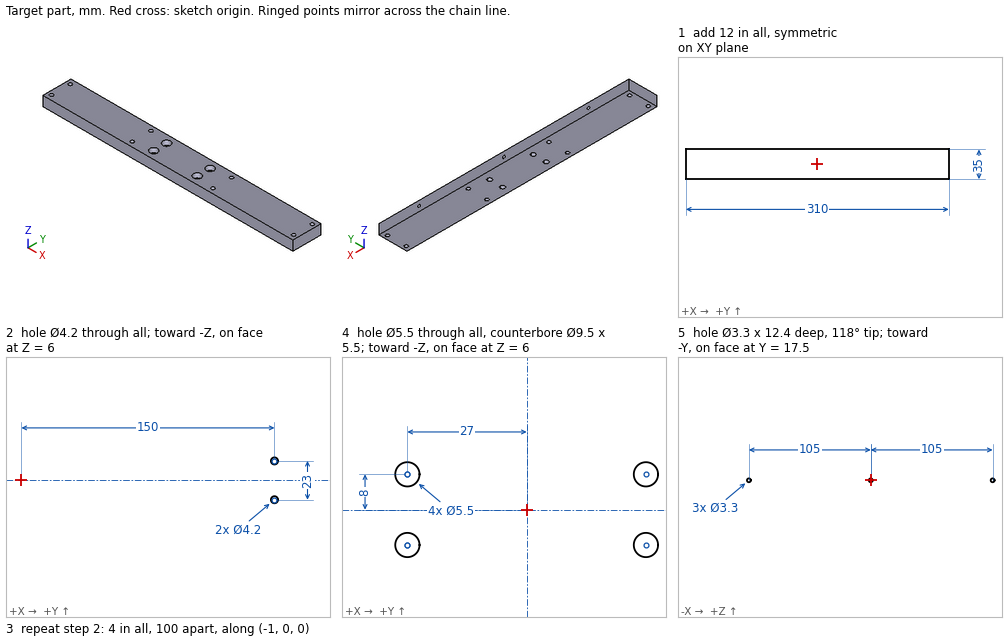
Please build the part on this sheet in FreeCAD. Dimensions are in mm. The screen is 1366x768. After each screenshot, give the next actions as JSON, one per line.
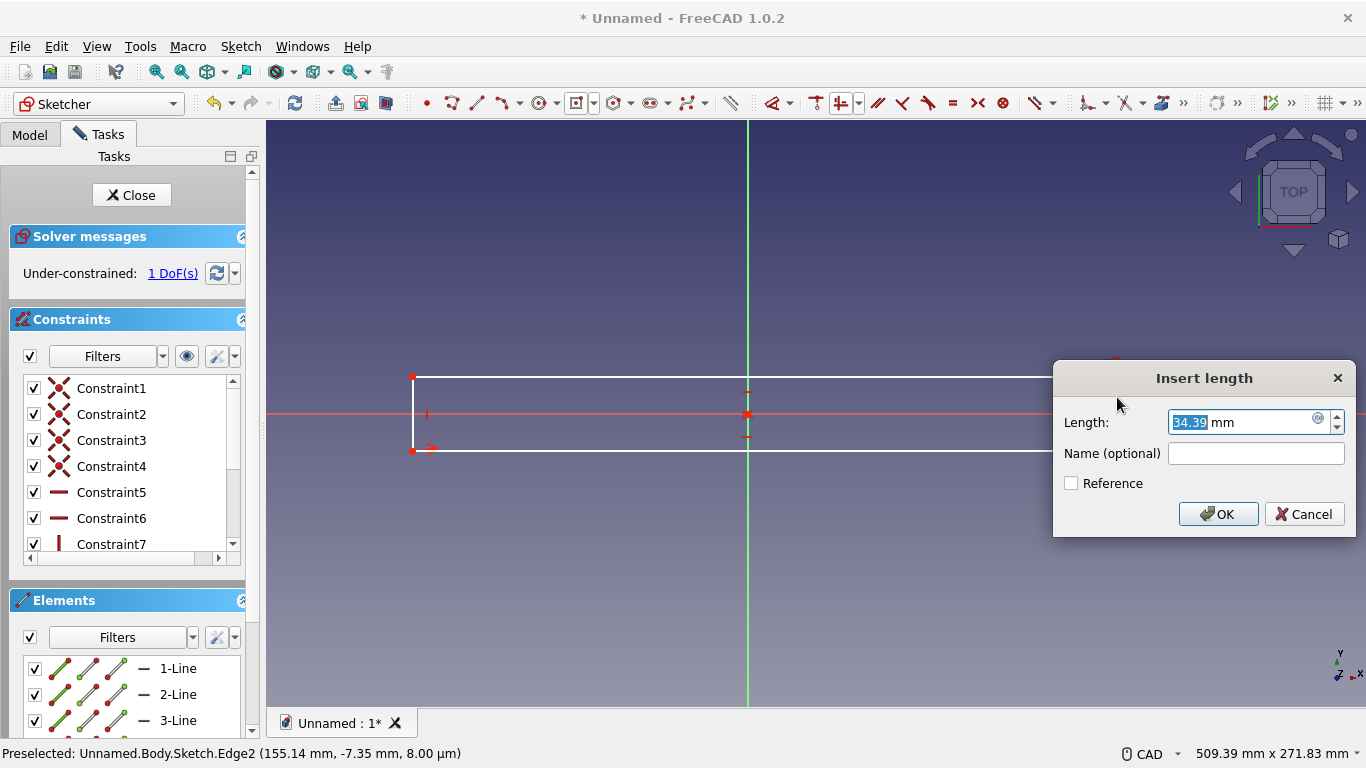
{"action": "type", "text": "35"}
{"action": "key", "text": "Return"}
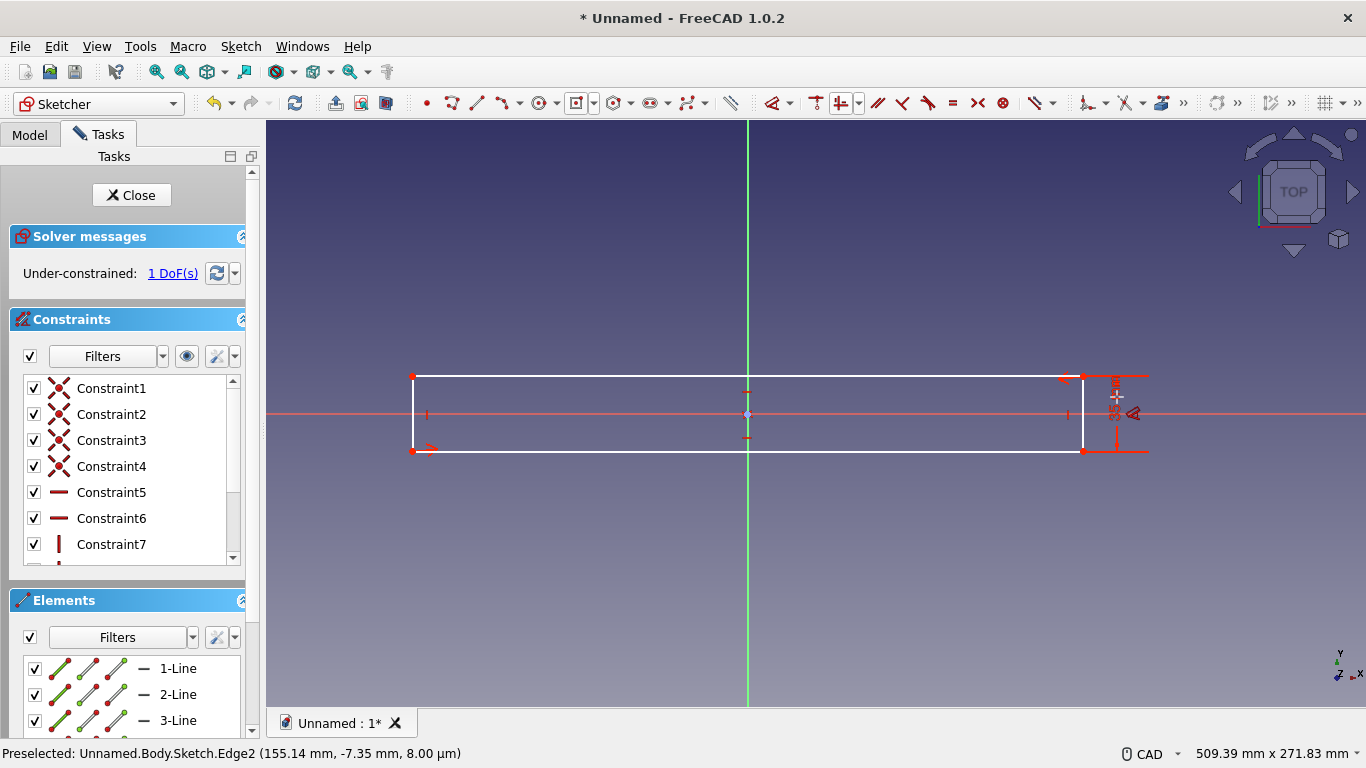
{"action": "left_click", "coordinate": [614, 452]}
{"action": "left_click", "coordinate": [594, 486]}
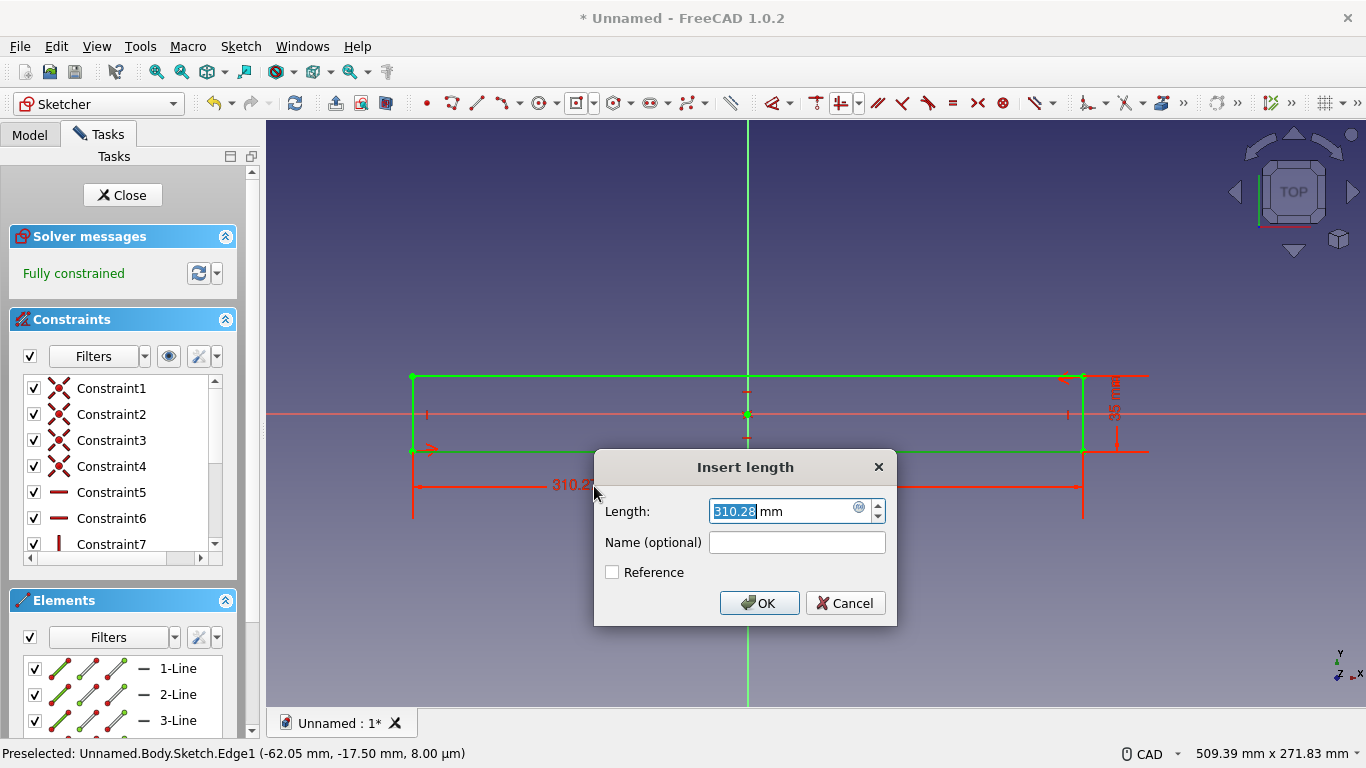
{"action": "type", "text": "310"}
{"action": "key", "text": "Return"}
{"action": "key", "text": "Escape"}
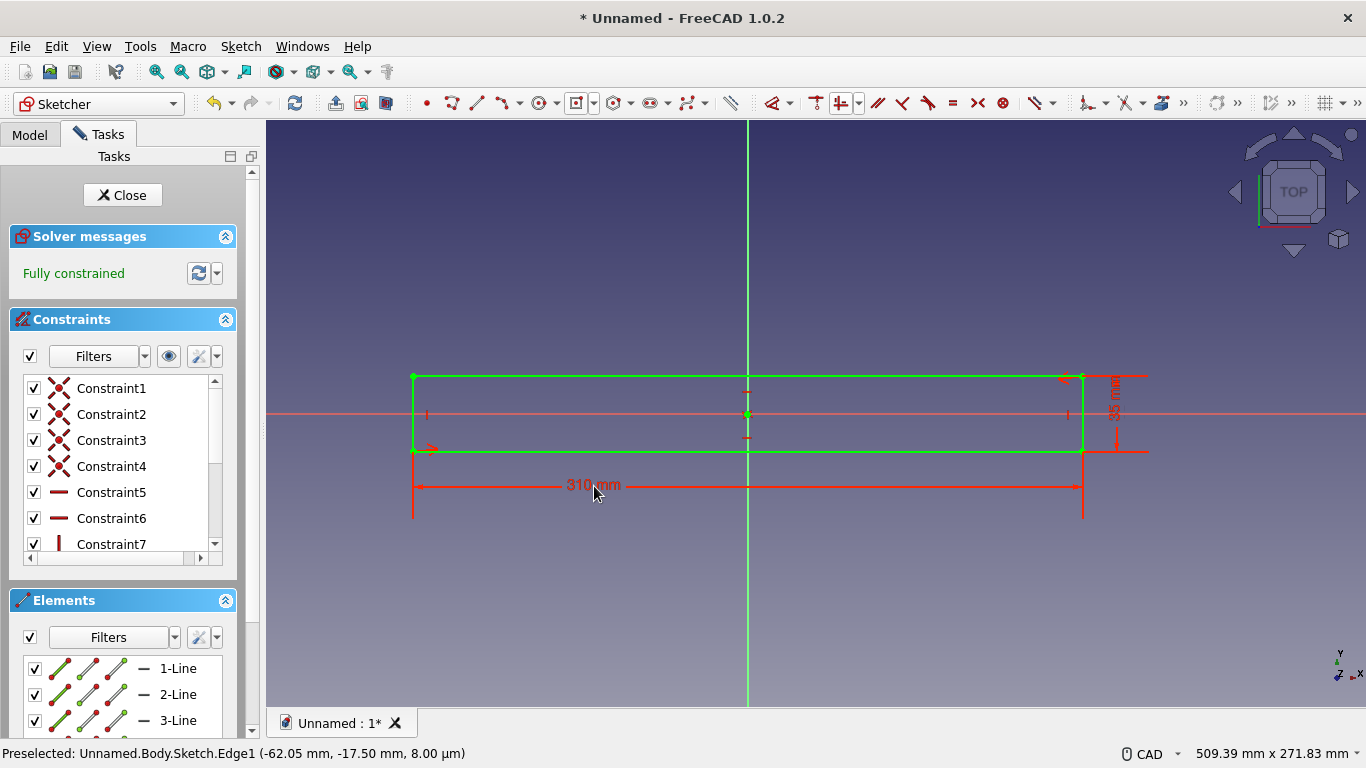
{"action": "left_click", "coordinate": [123, 195]}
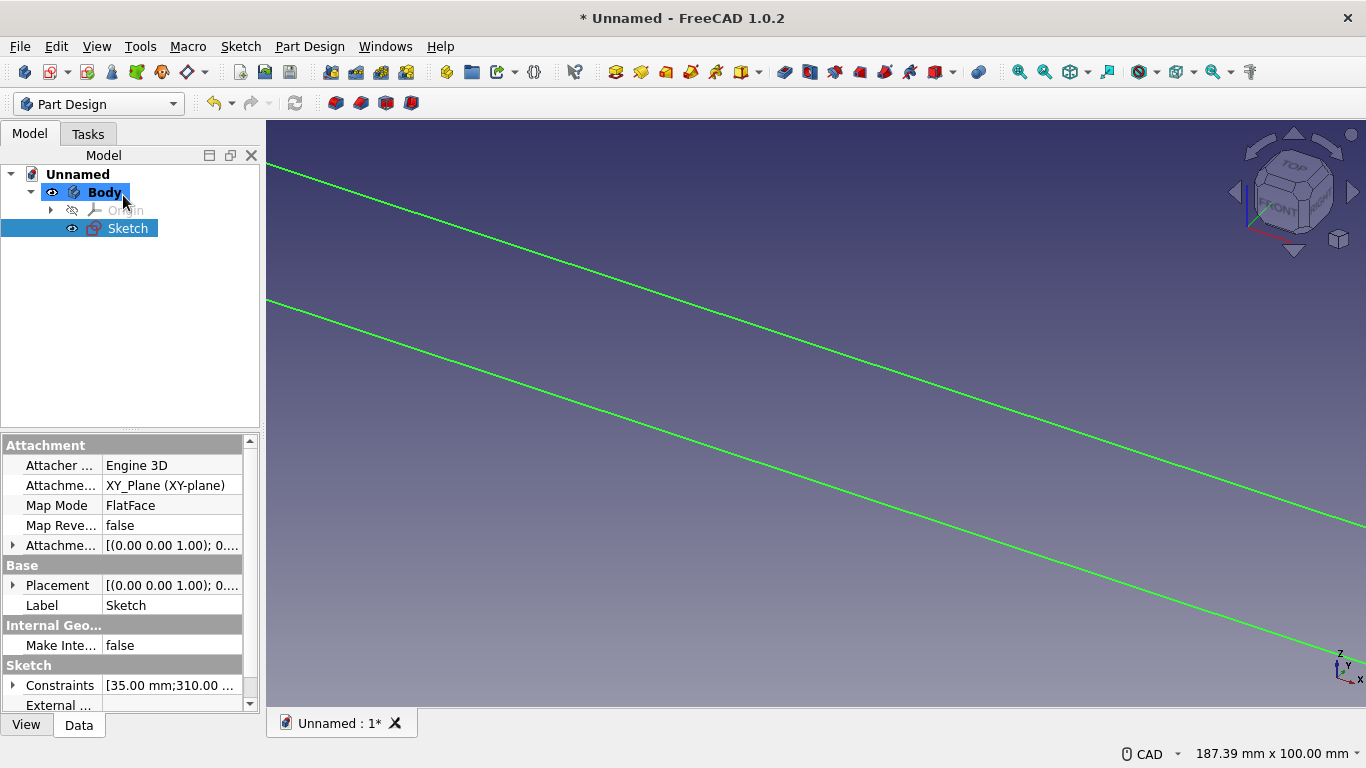
{"action": "left_click", "coordinate": [616, 72]}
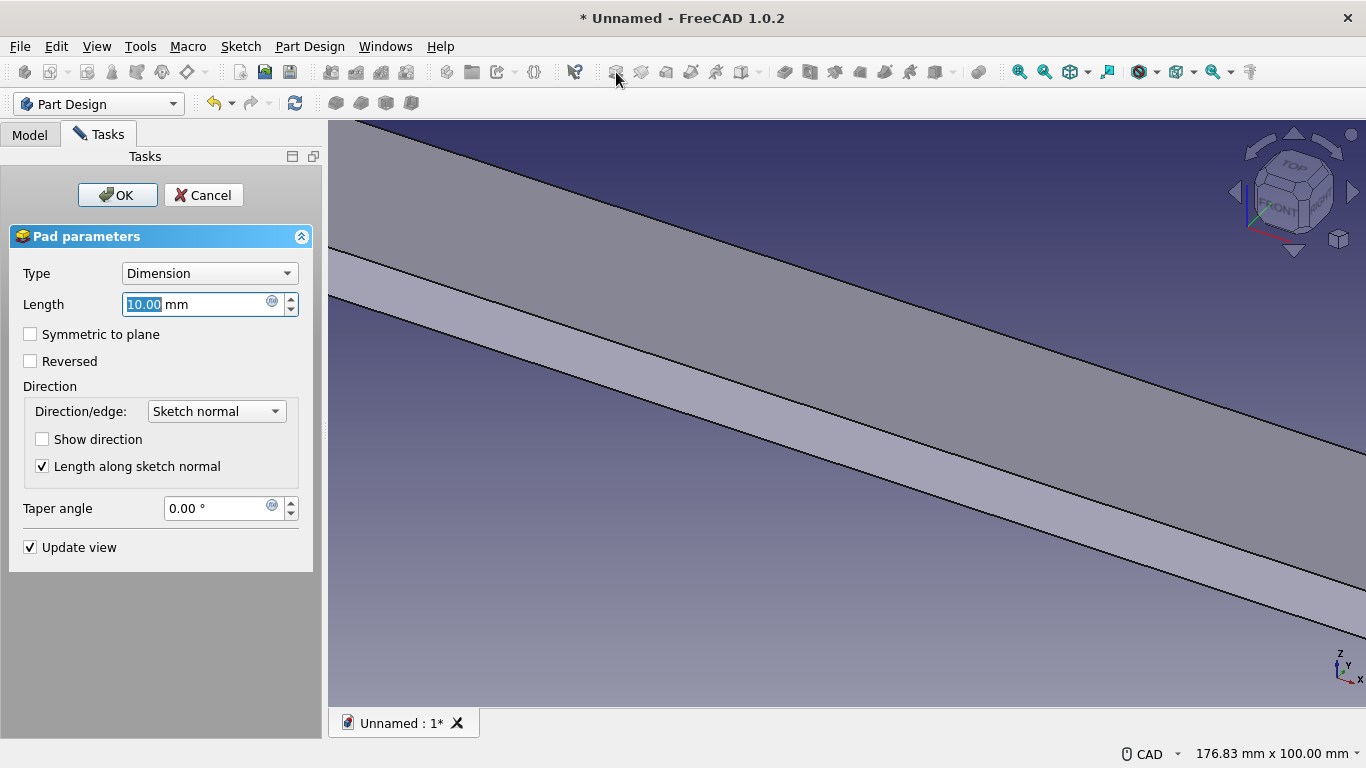
{"action": "type", "text": "12"}
{"action": "key", "text": "Tab"}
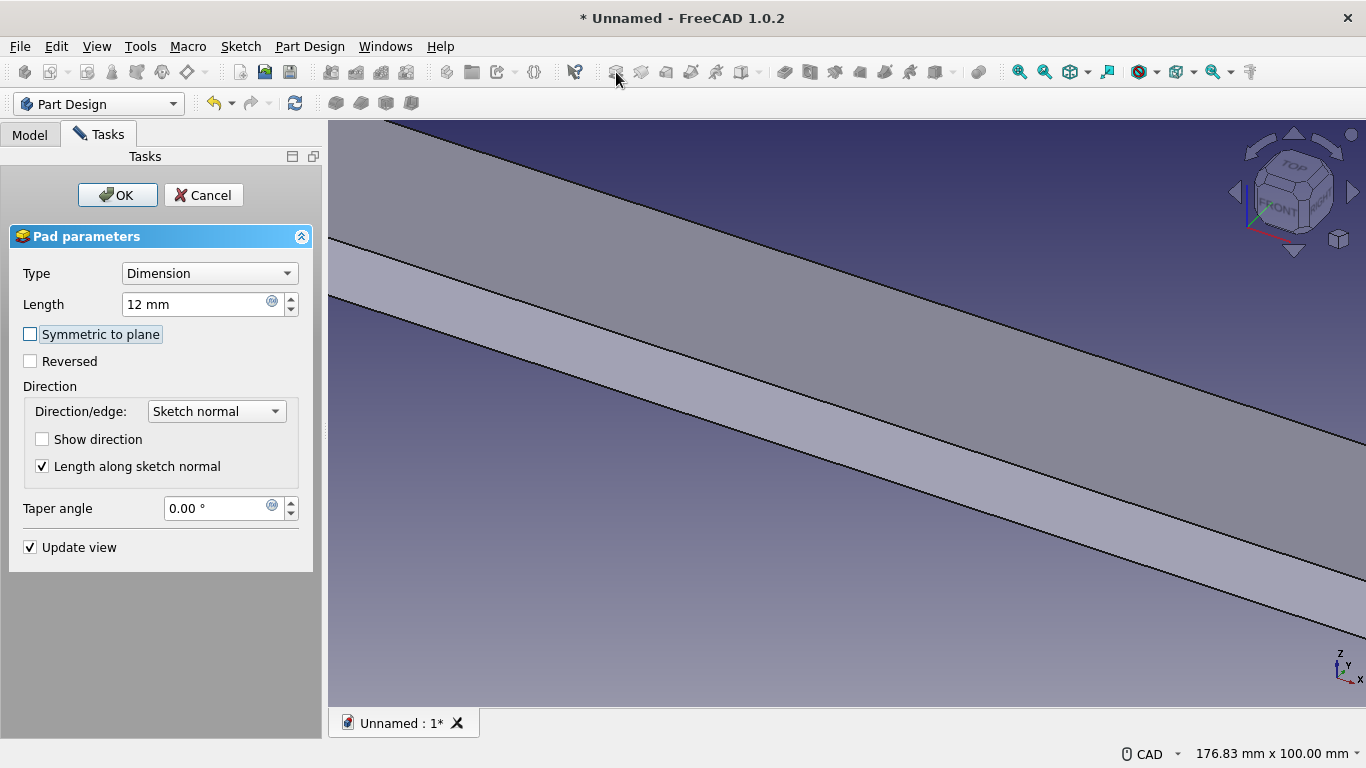
{"action": "left_click", "coordinate": [31, 334]}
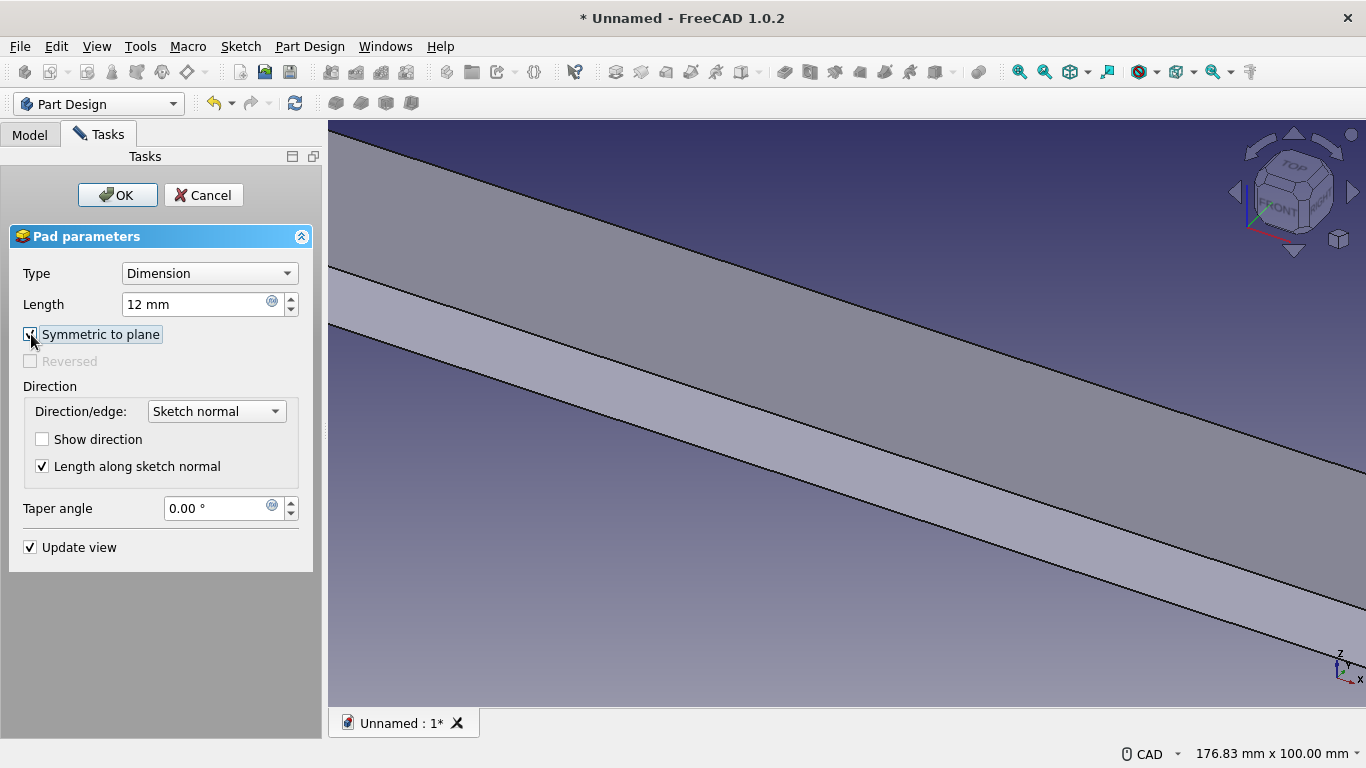
{"action": "left_click", "coordinate": [118, 195]}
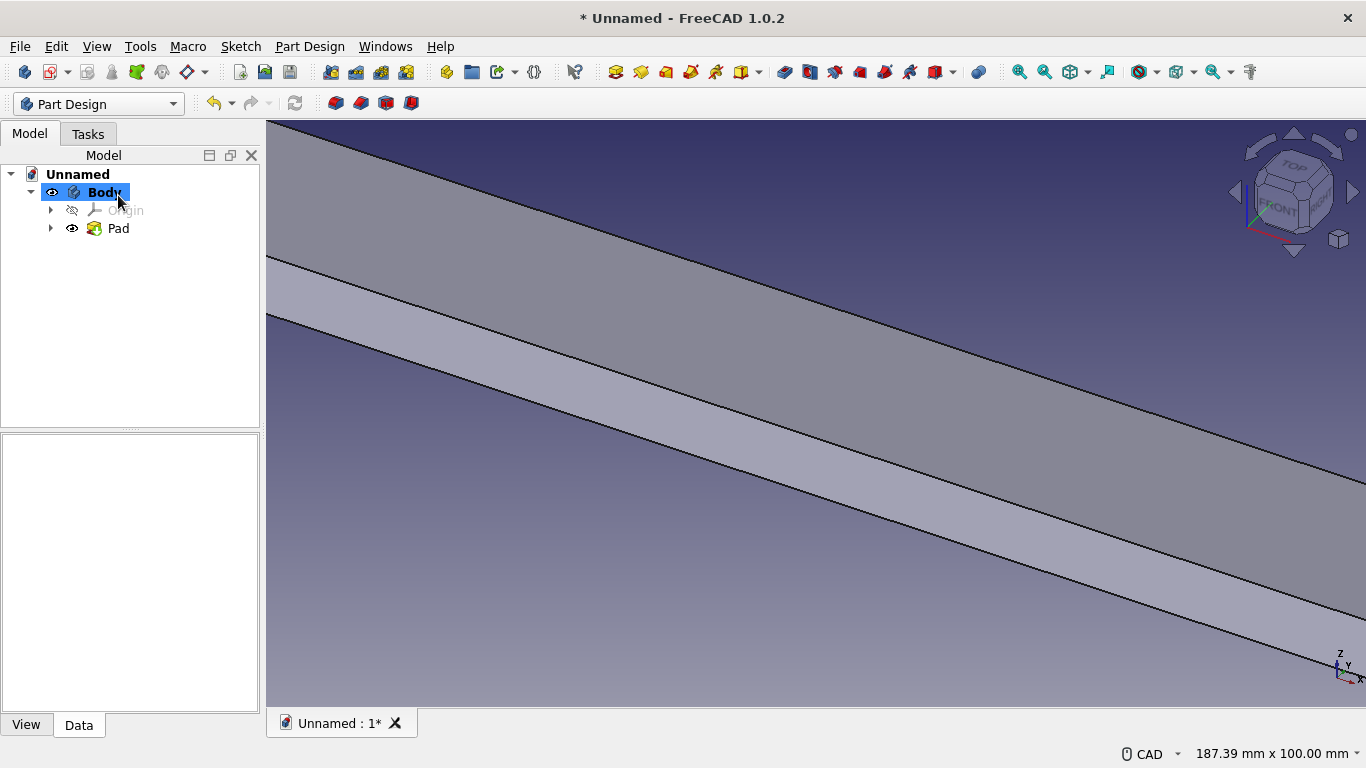
{"action": "left_click", "coordinate": [1020, 72]}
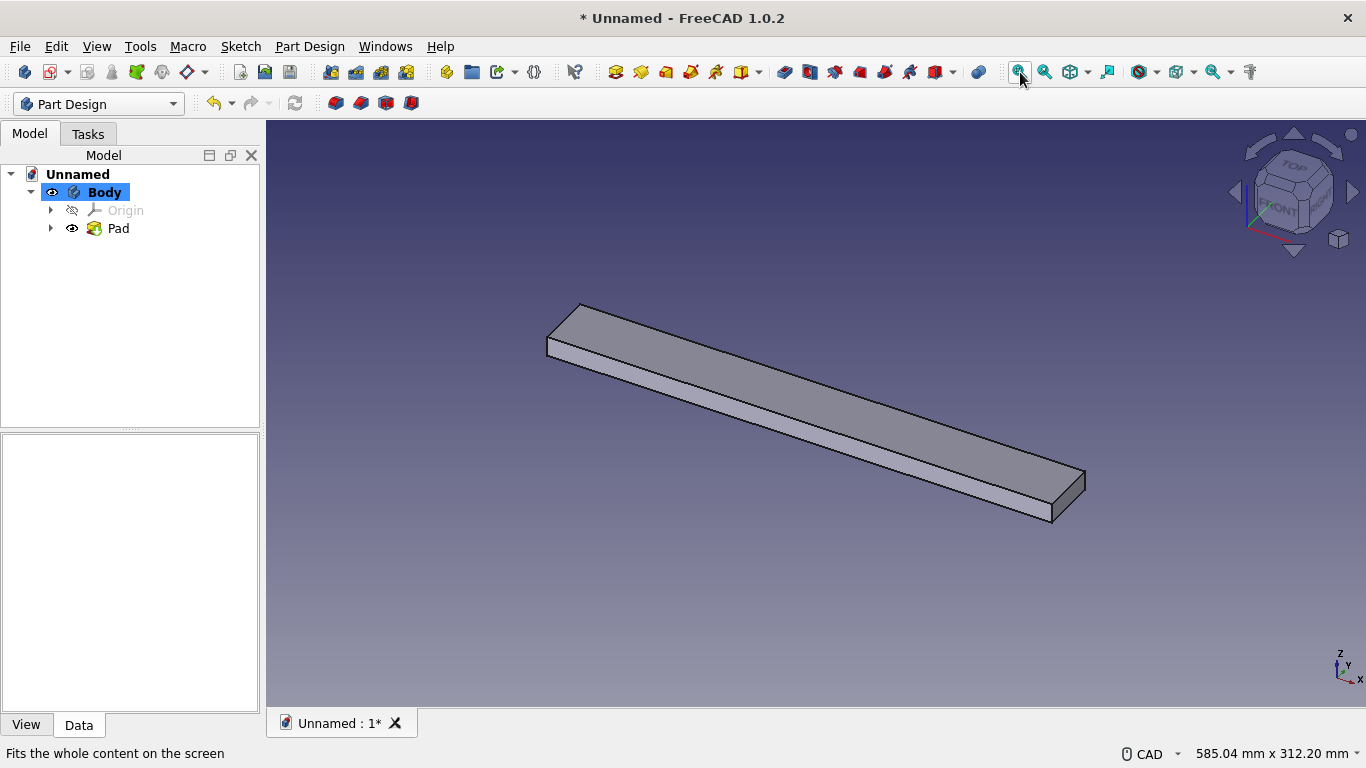
{"action": "left_click", "coordinate": [1032, 475]}